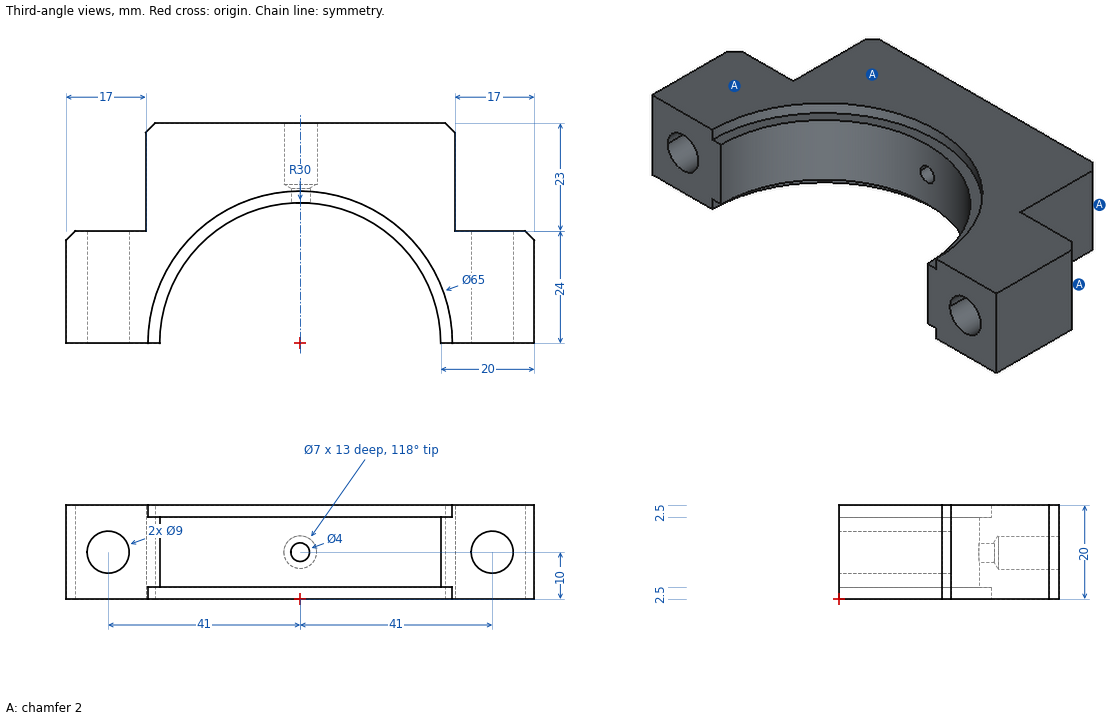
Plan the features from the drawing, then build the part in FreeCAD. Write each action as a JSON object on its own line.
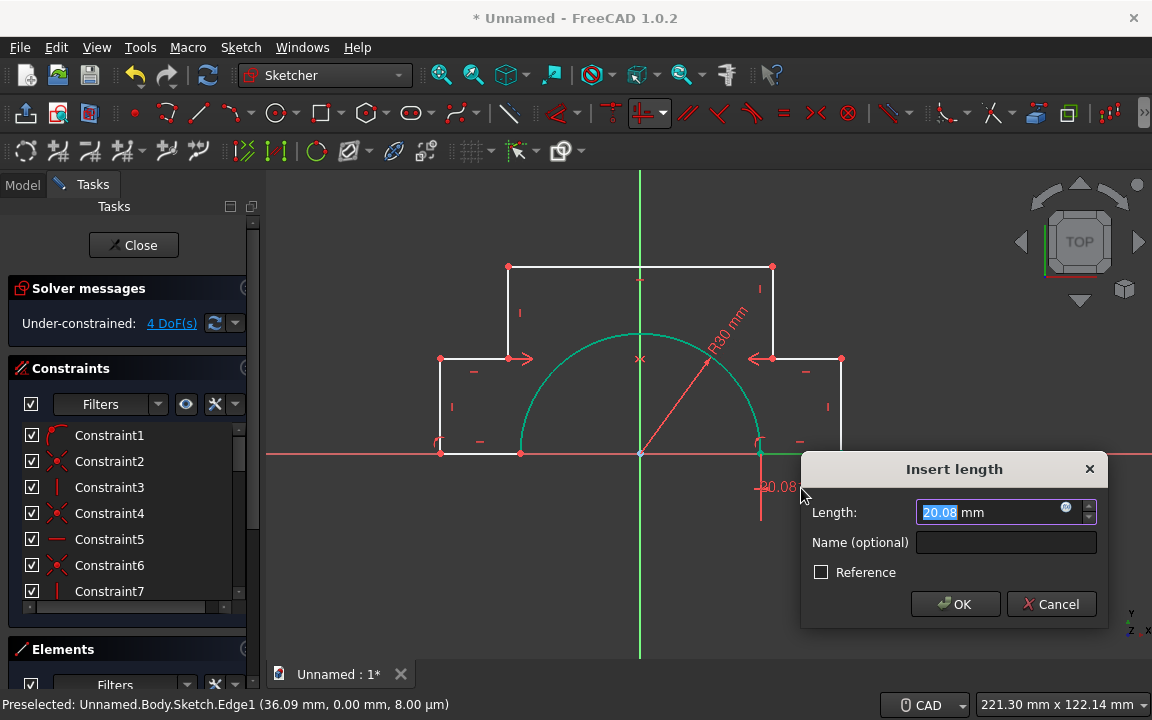
{"action": "type", "text": "20"}
{"action": "key", "text": "Return"}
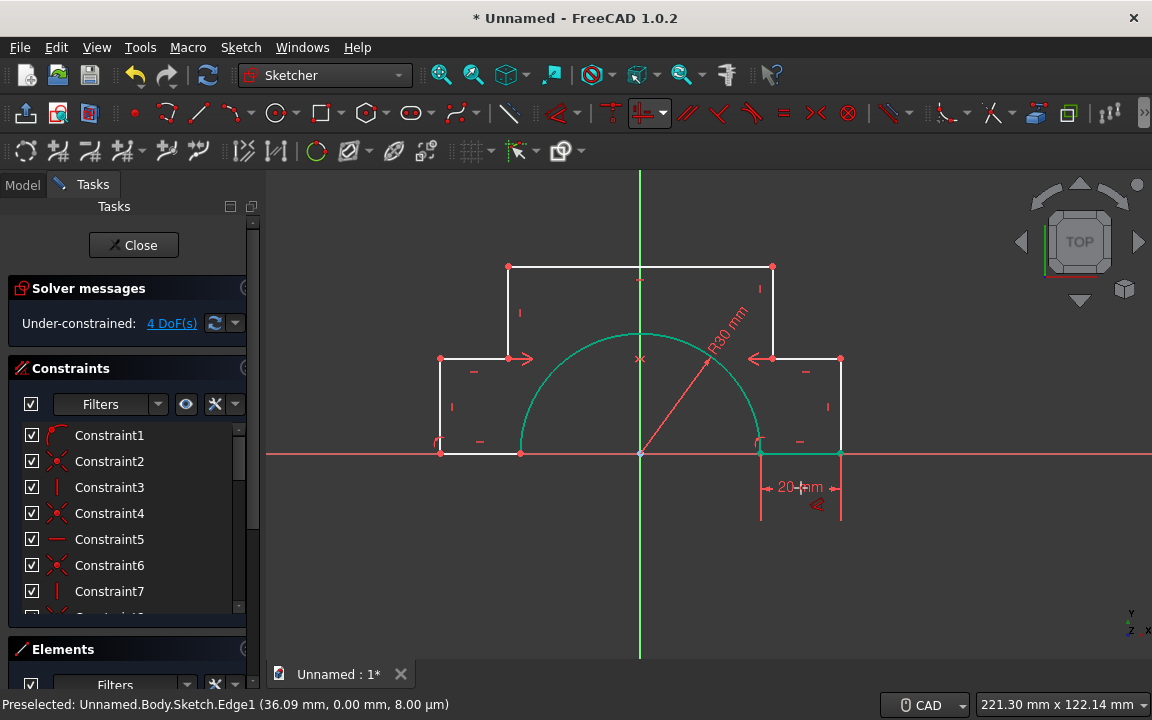
{"action": "left_click", "coordinate": [841, 425]}
{"action": "left_click", "coordinate": [875, 406]}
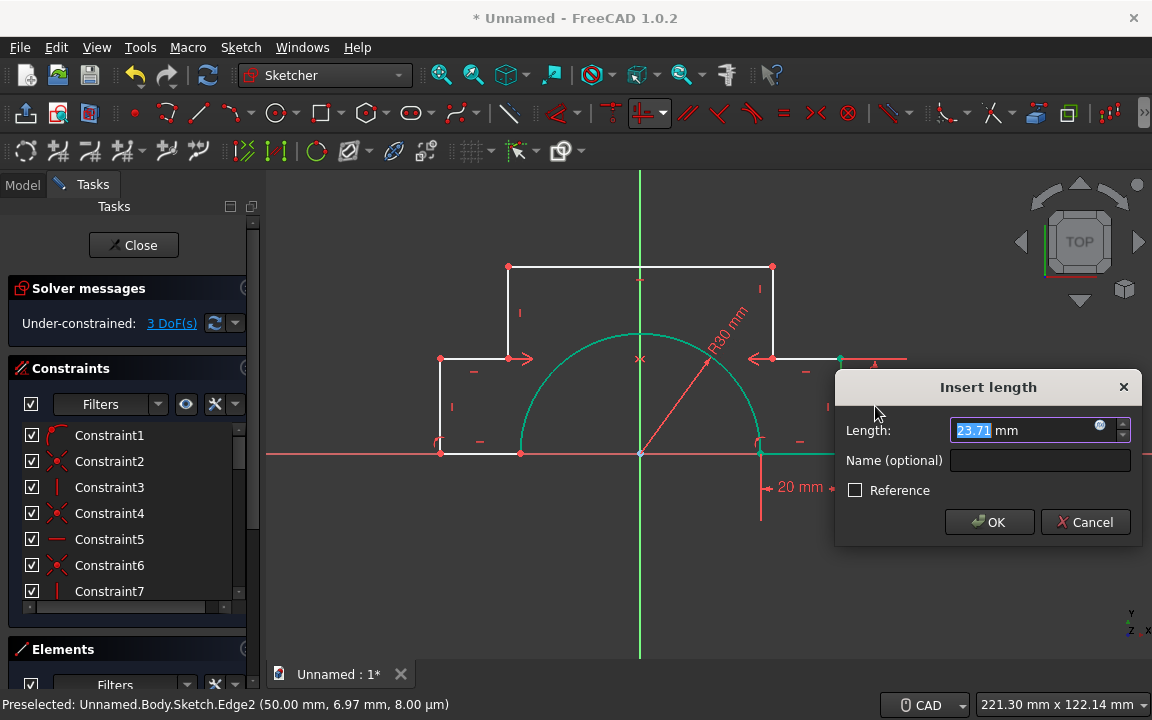
{"action": "type", "text": "24"}
{"action": "key", "text": "Return"}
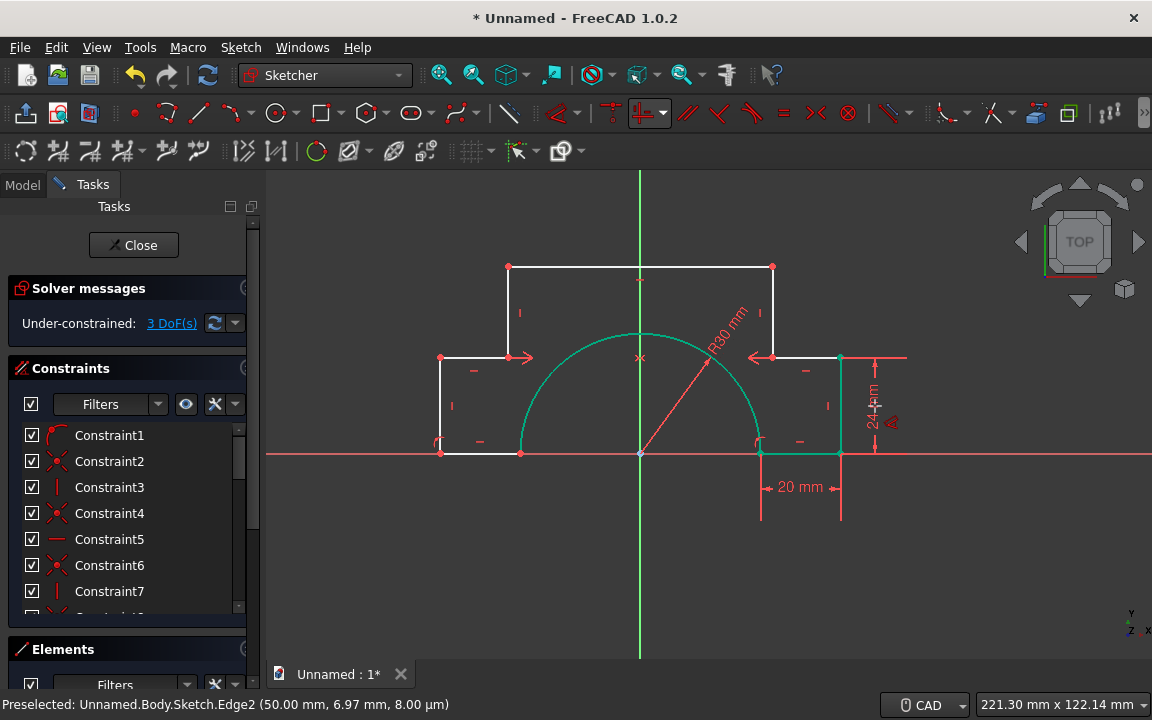
{"action": "left_click", "coordinate": [820, 358]}
{"action": "left_click", "coordinate": [807, 324]}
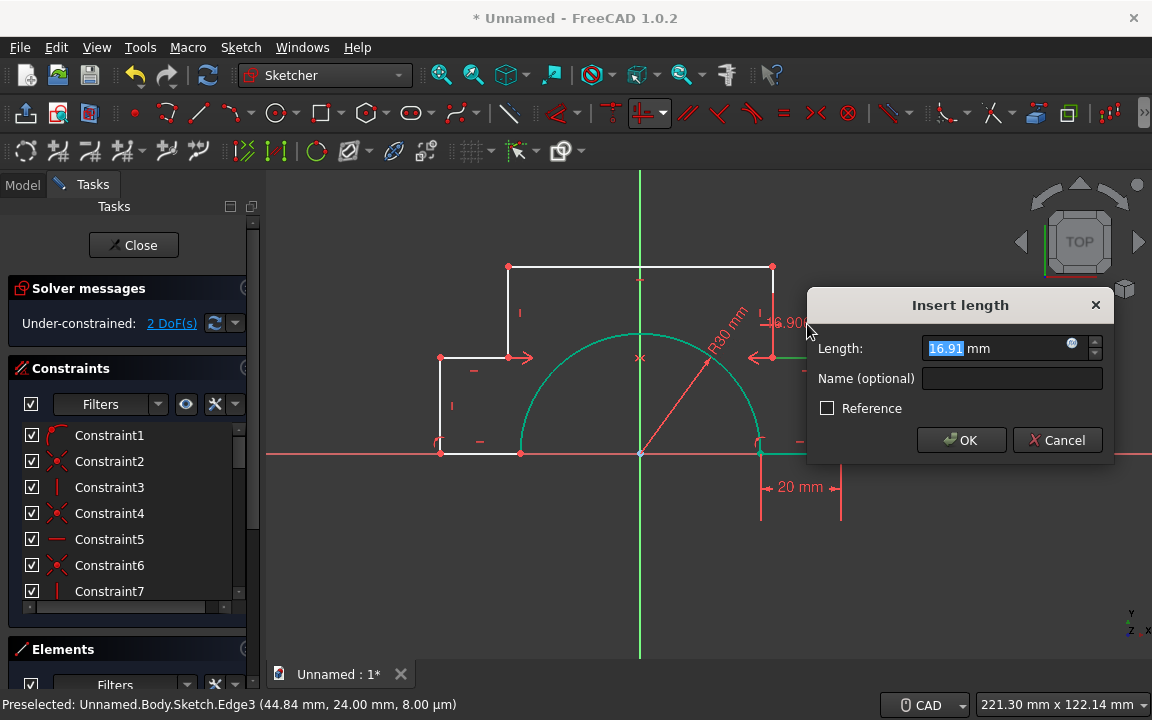
{"action": "type", "text": "17"}
{"action": "key", "text": "Return"}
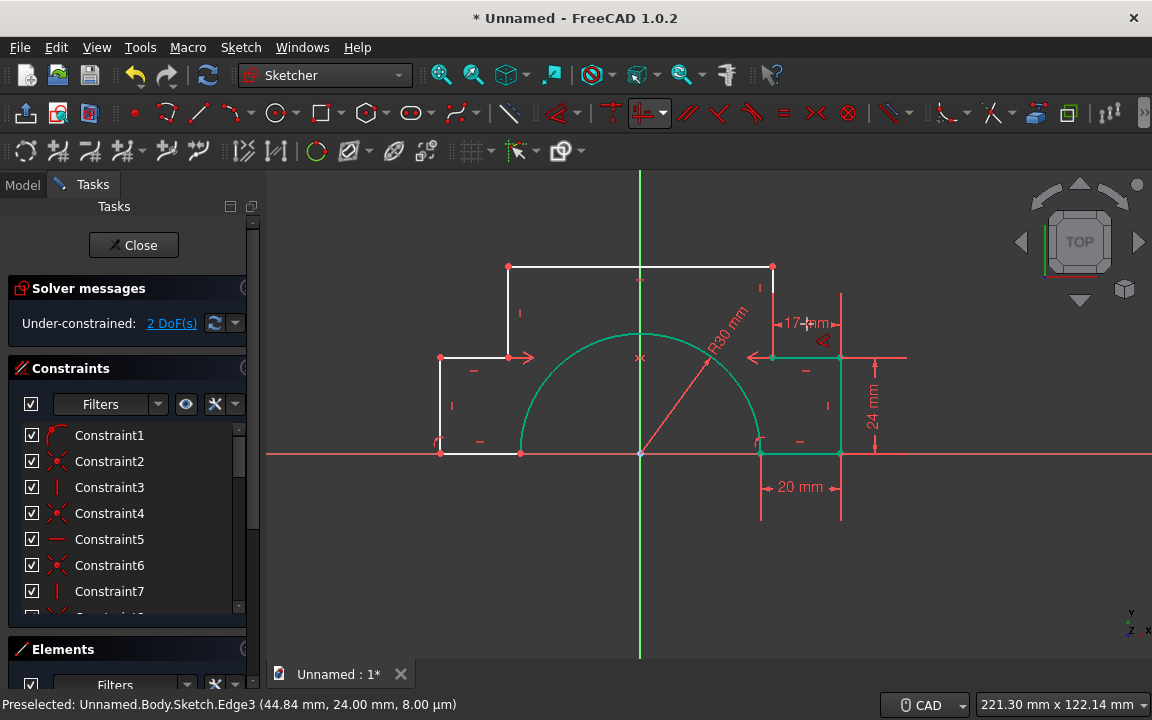
{"action": "left_click", "coordinate": [773, 331]}
{"action": "left_click", "coordinate": [807, 292]}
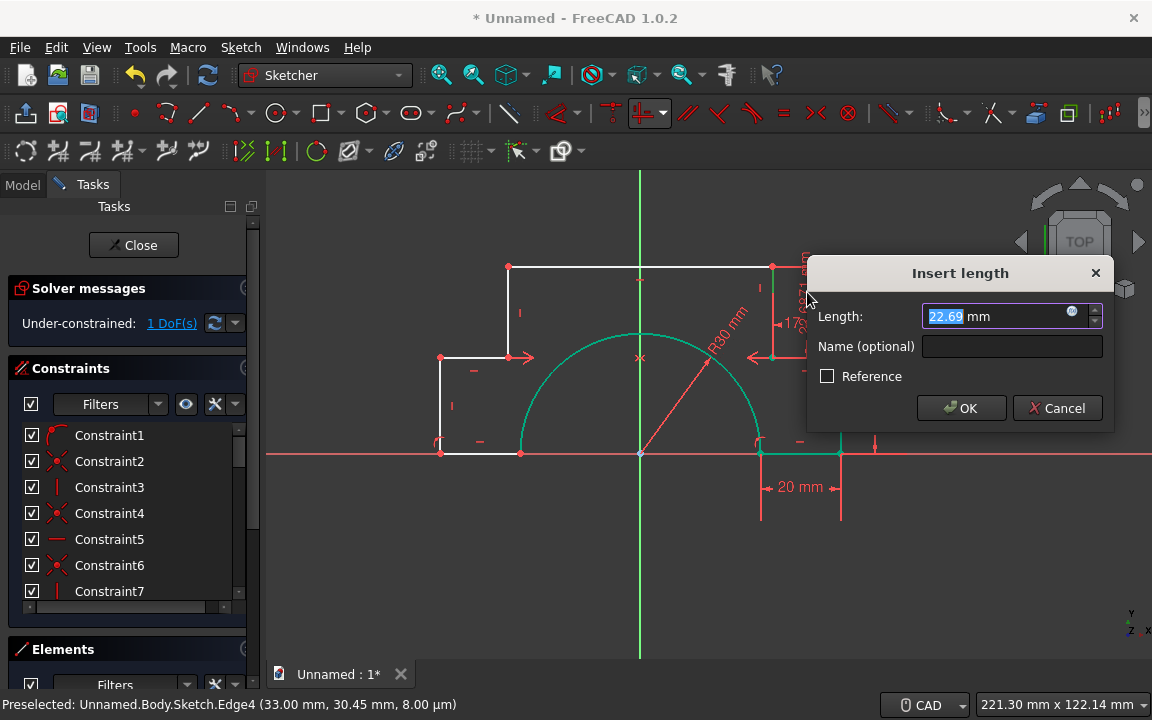
{"action": "type", "text": "23"}
{"action": "key", "text": "Return"}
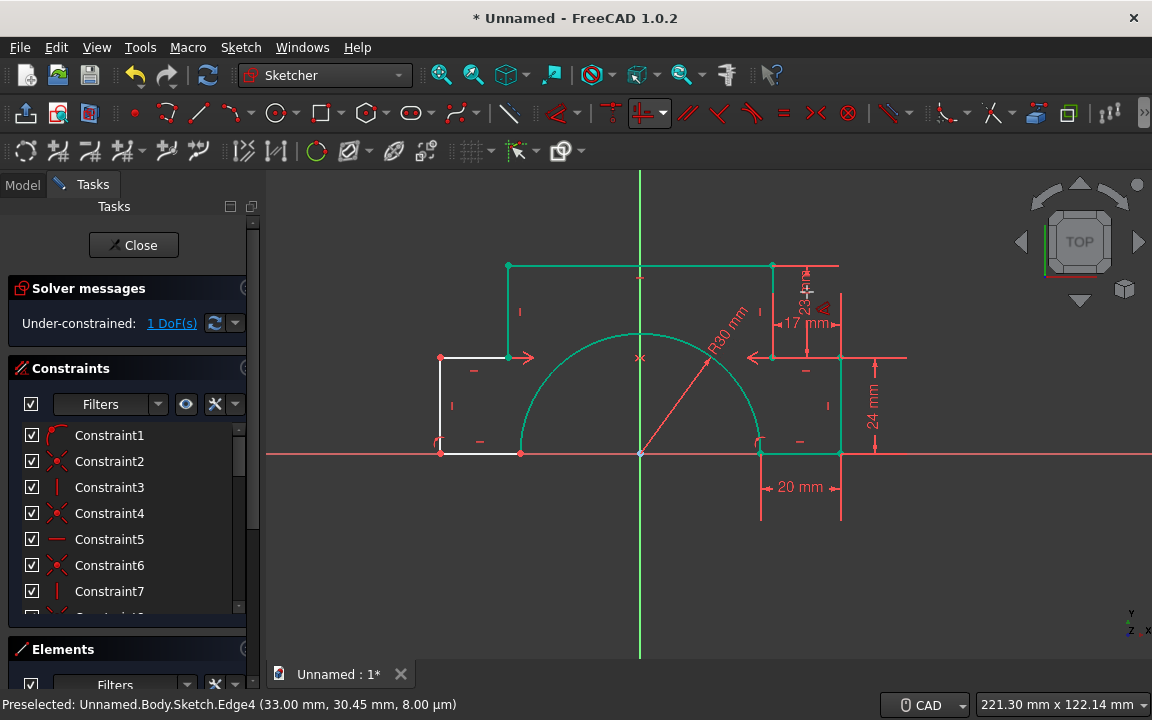
{"action": "left_click", "coordinate": [488, 358]}
{"action": "left_click", "coordinate": [474, 324]}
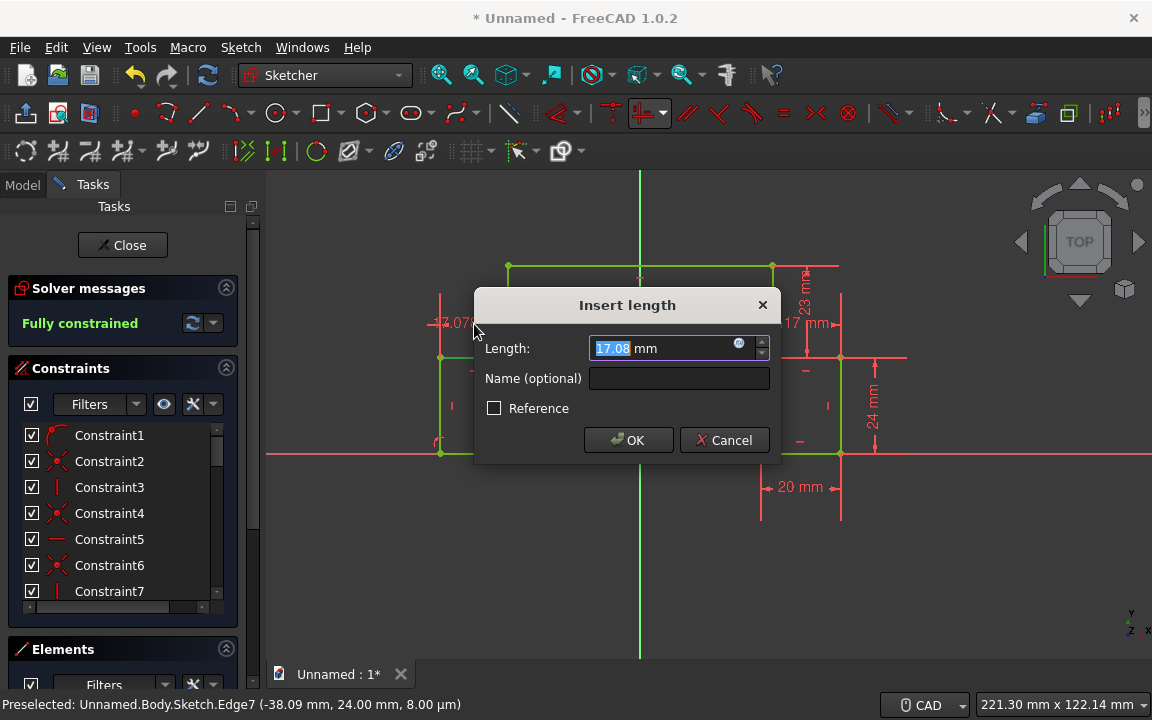
{"action": "type", "text": "17"}
{"action": "key", "text": "Return"}
{"action": "key", "text": "Escape"}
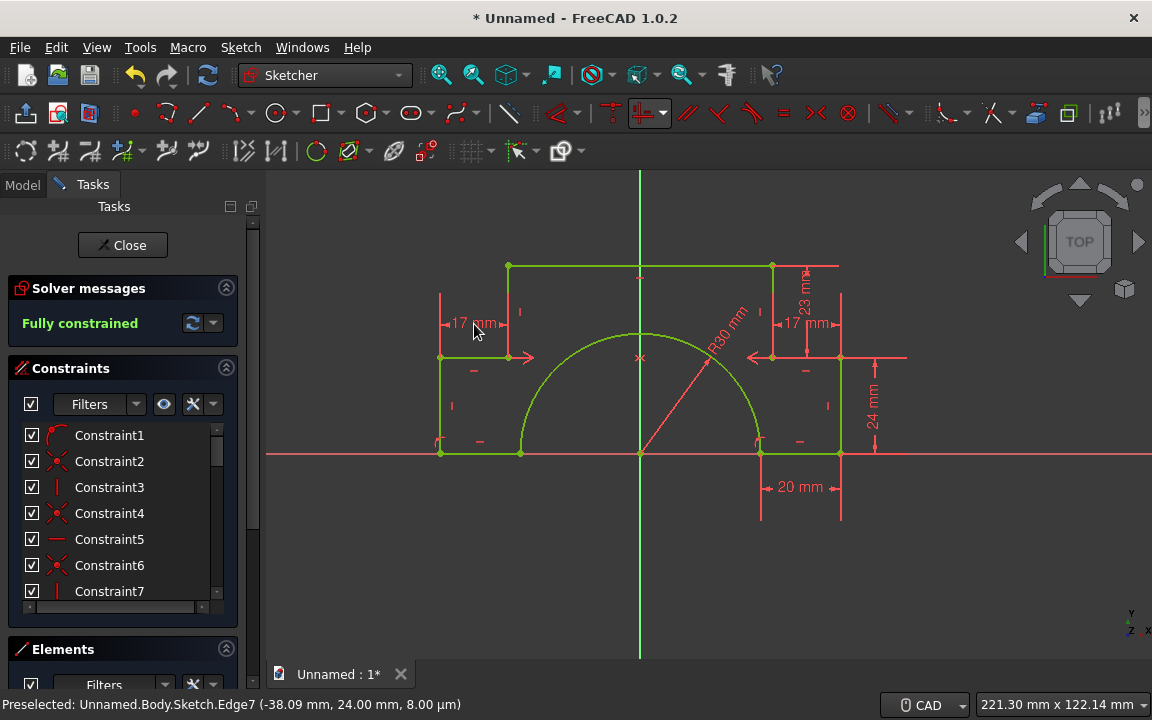
{"action": "left_click", "coordinate": [123, 245]}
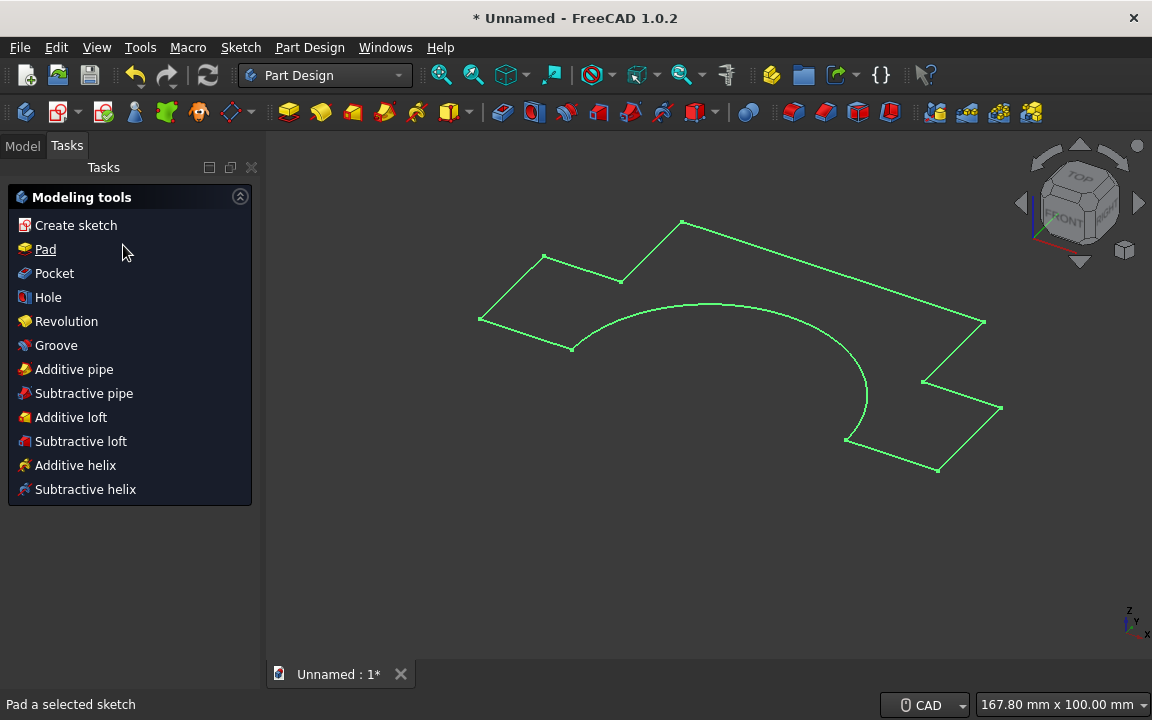
{"action": "left_click", "coordinate": [290, 112]}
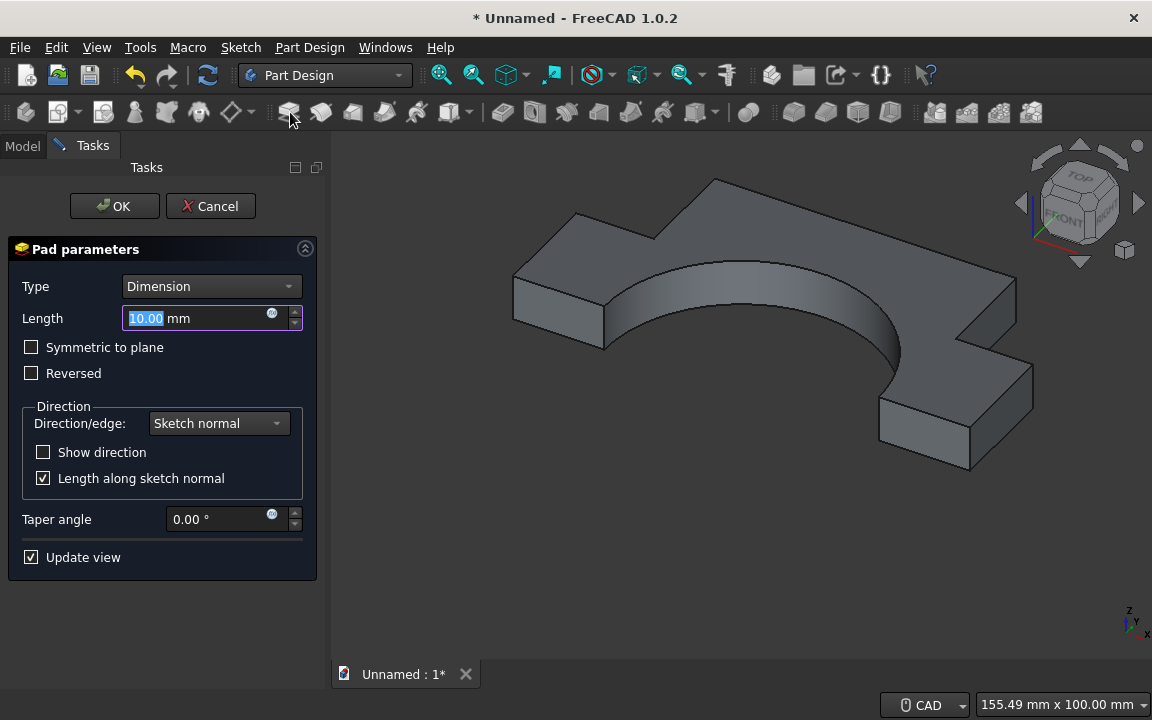
{"action": "type", "text": "20"}
{"action": "key", "text": "Tab"}